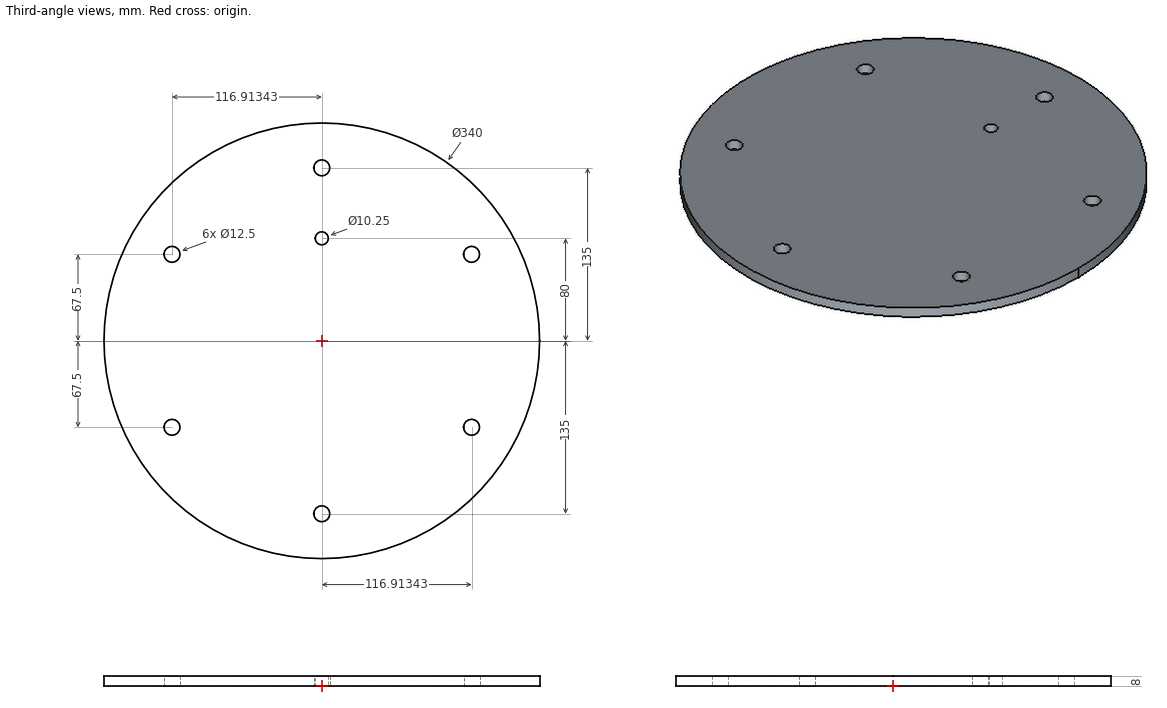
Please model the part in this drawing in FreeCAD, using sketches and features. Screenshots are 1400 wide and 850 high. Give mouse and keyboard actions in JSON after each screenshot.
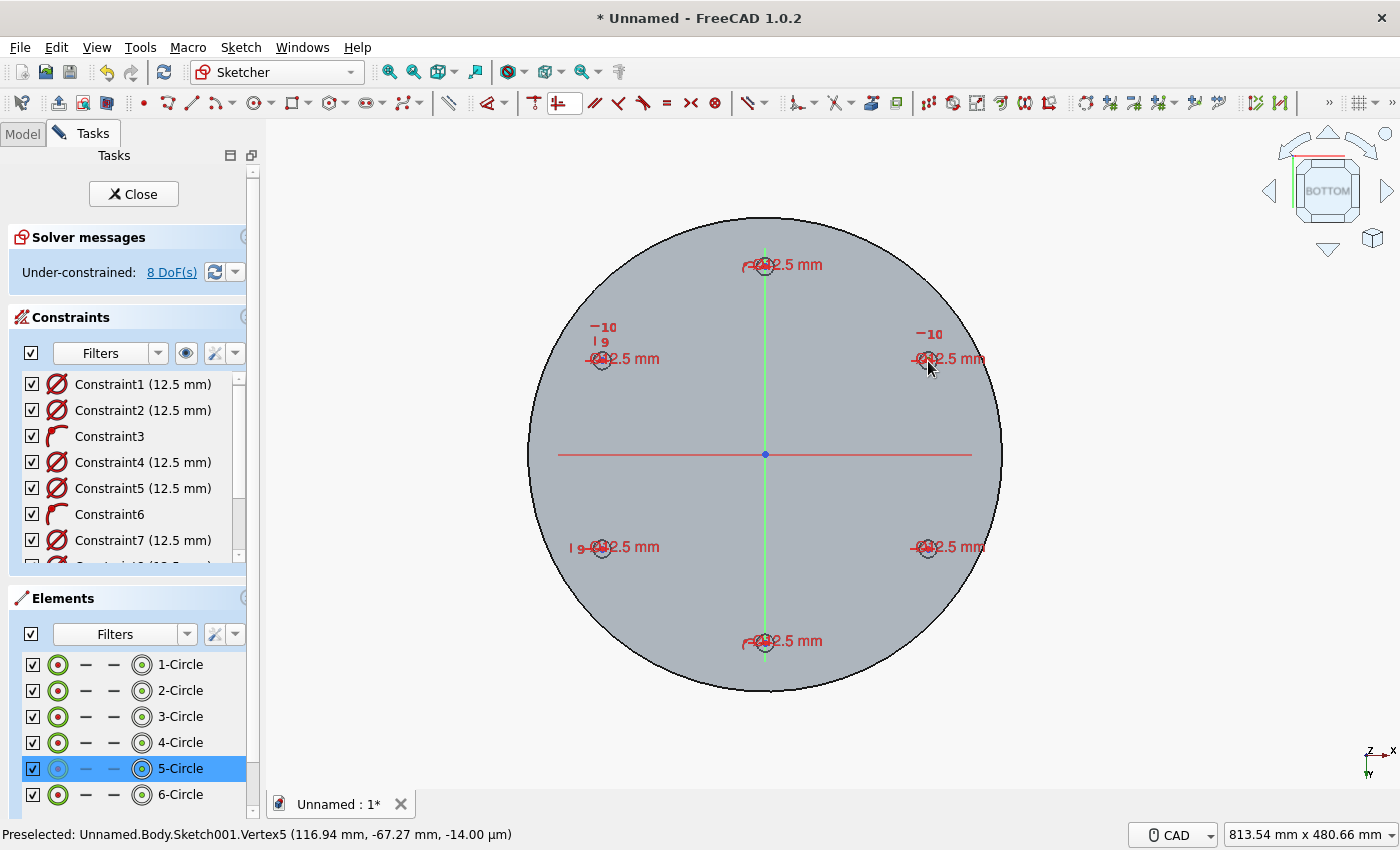
{"action": "left_click", "coordinate": [928, 549]}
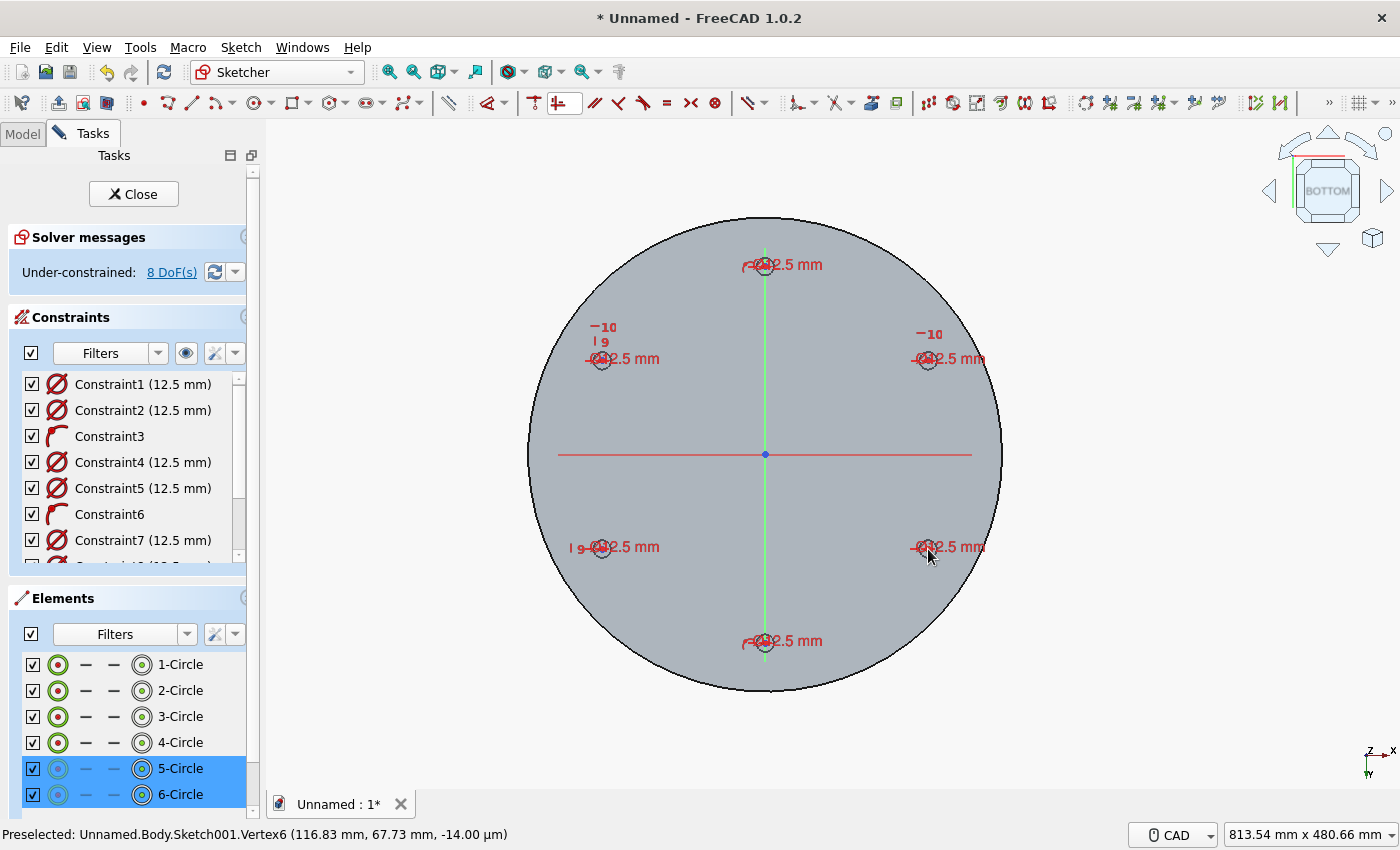
{"action": "key", "text": "v"}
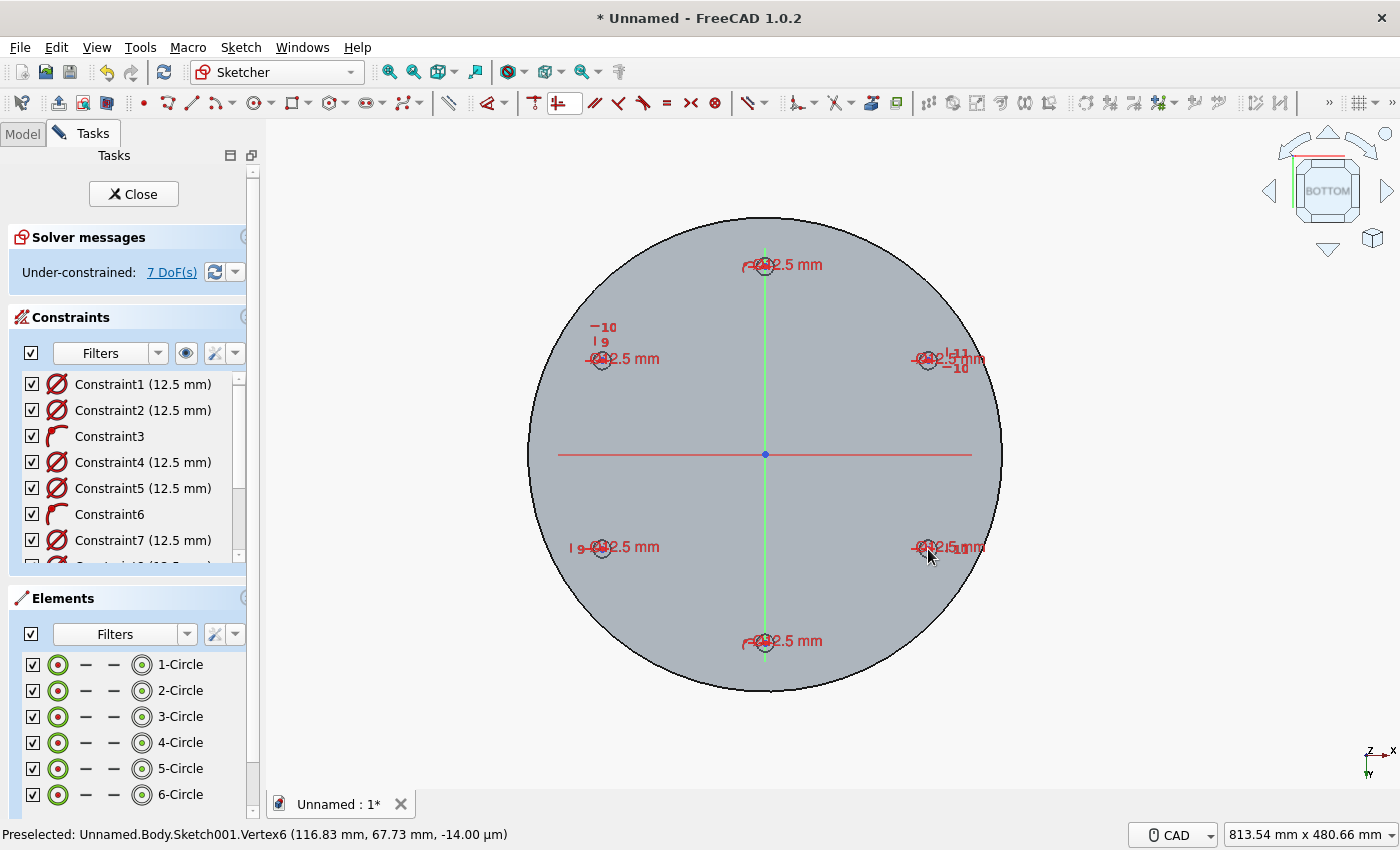
{"action": "left_click", "coordinate": [602, 549]}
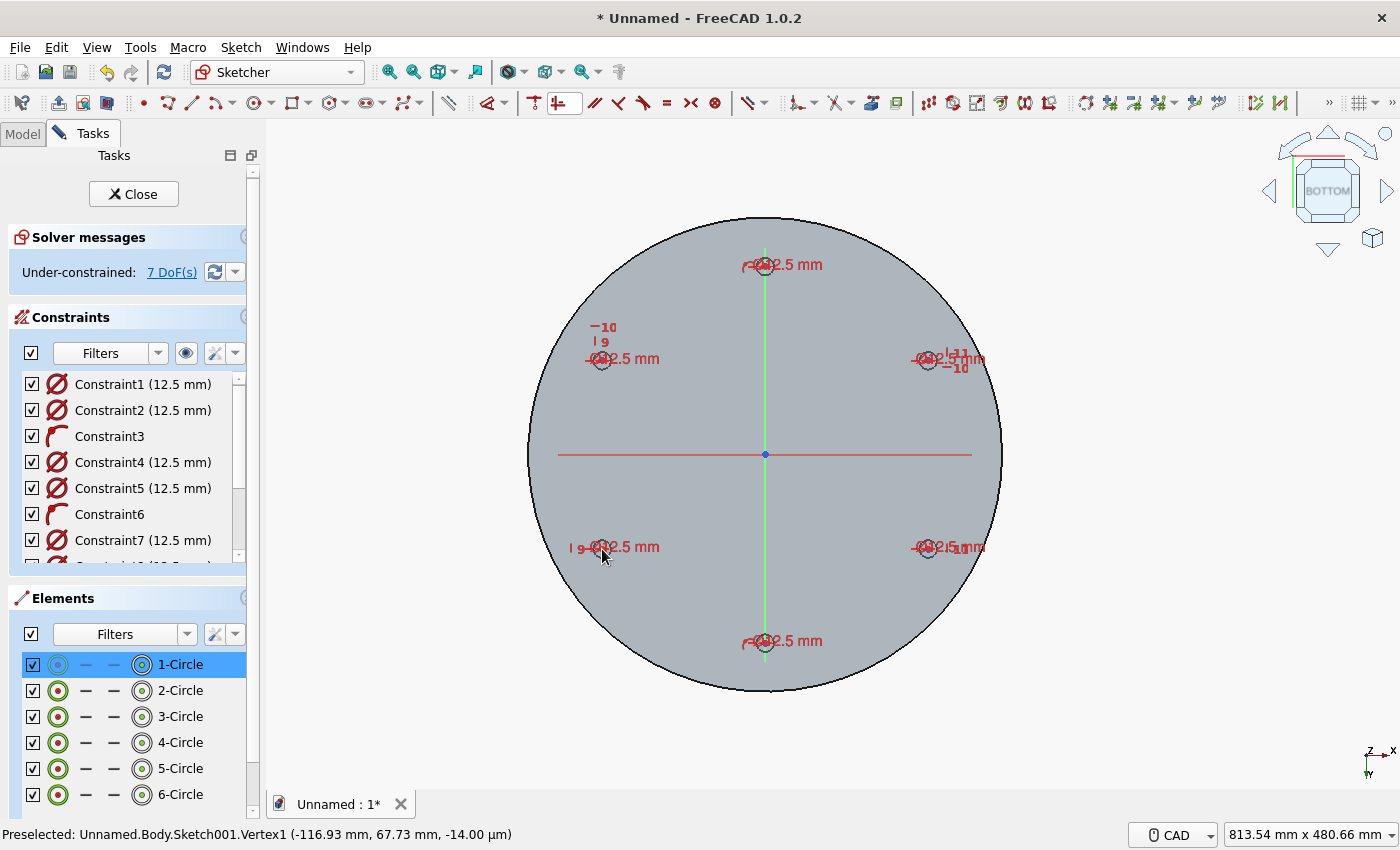
{"action": "left_click", "coordinate": [928, 549]}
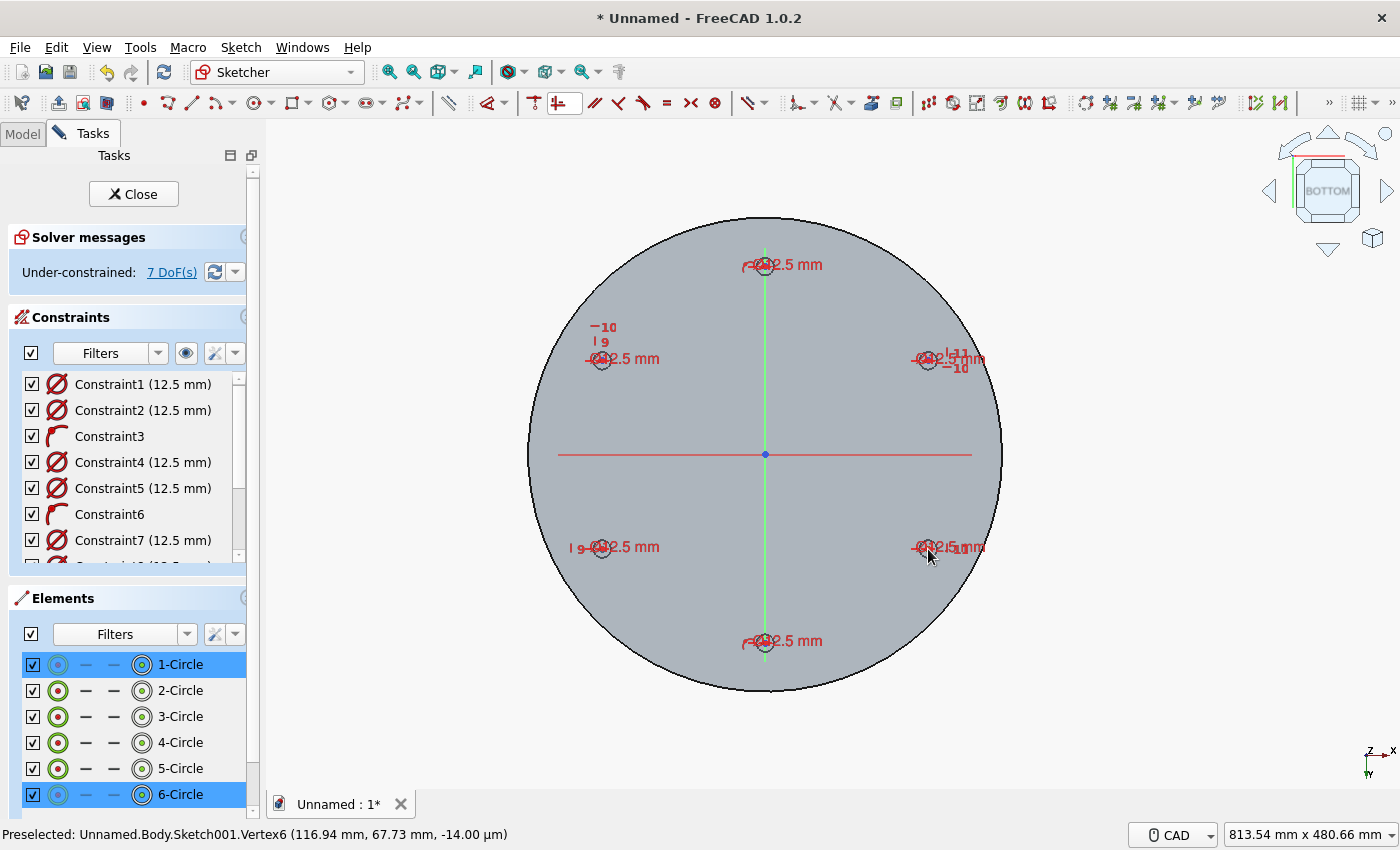
{"action": "key", "text": "h"}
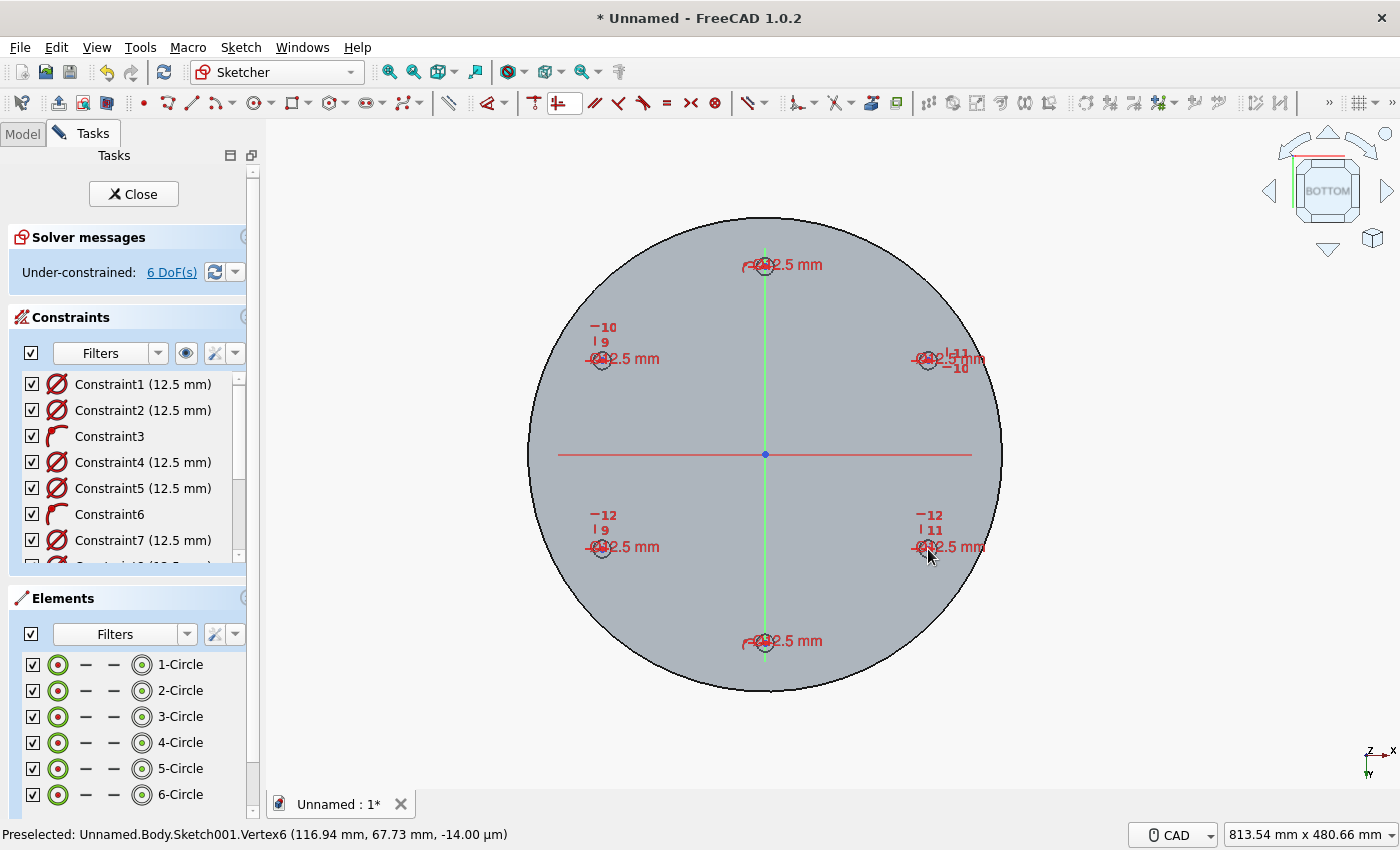
{"action": "left_click", "coordinate": [488, 104]}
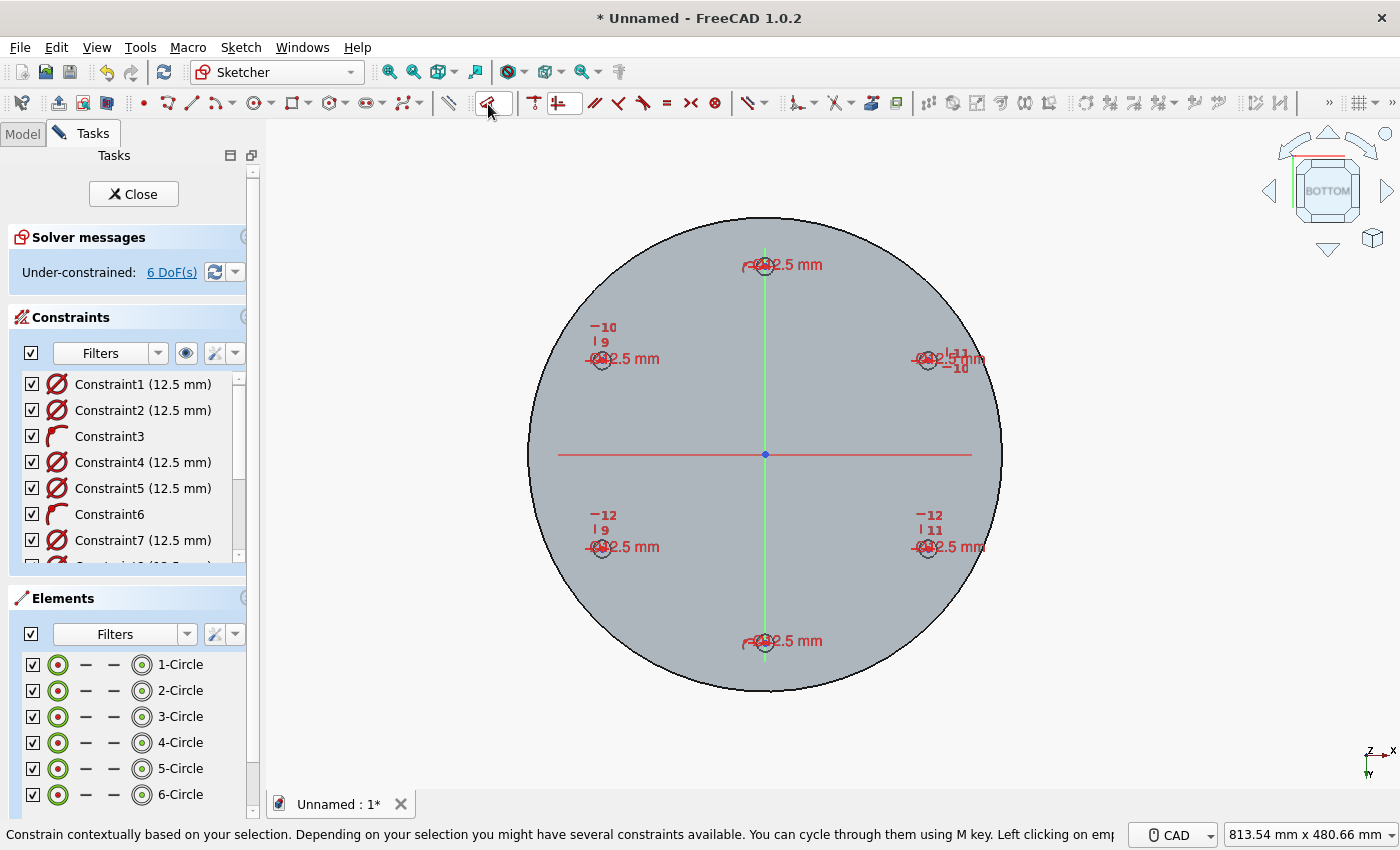
{"action": "left_click", "coordinate": [765, 643]}
{"action": "left_click", "coordinate": [799, 549]}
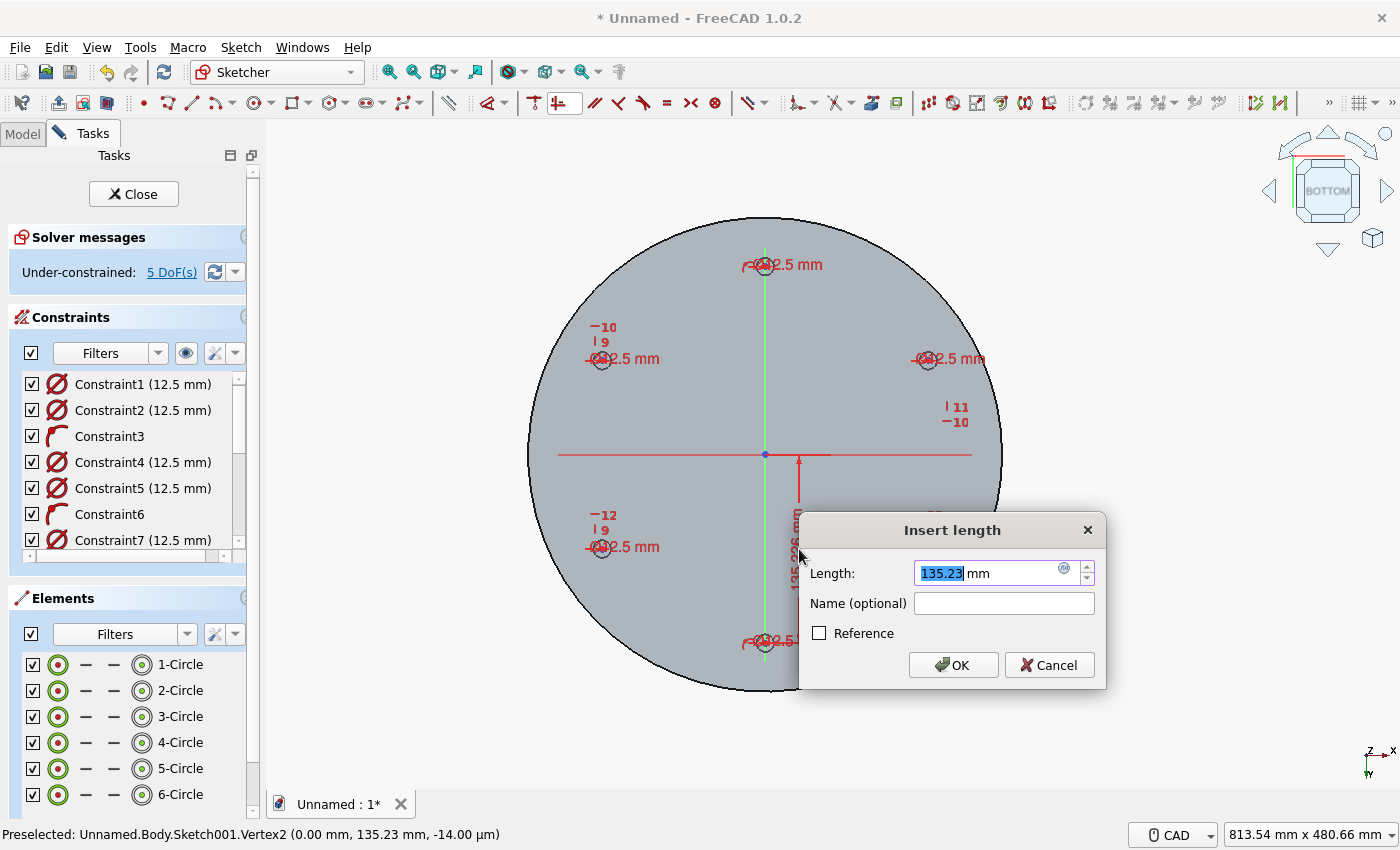
{"action": "type", "text": "135"}
{"action": "key", "text": "Return"}